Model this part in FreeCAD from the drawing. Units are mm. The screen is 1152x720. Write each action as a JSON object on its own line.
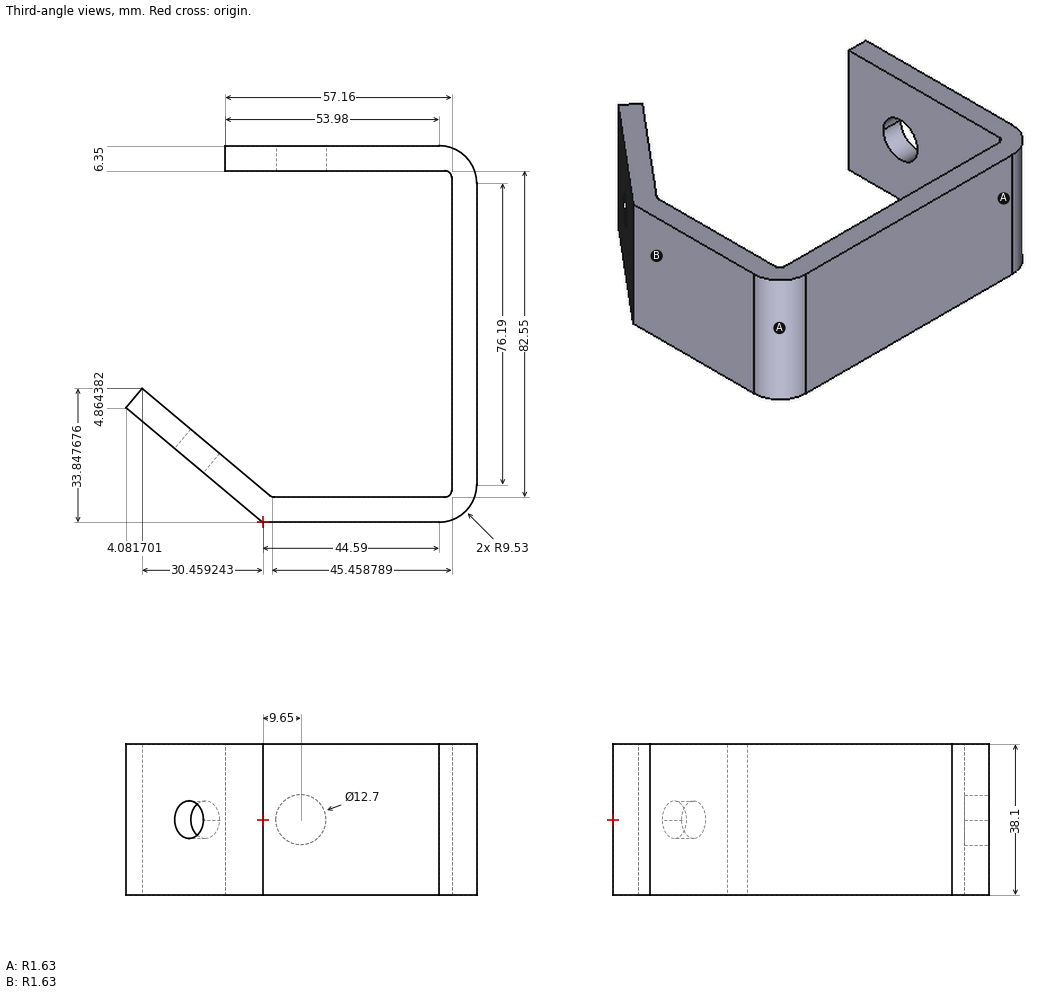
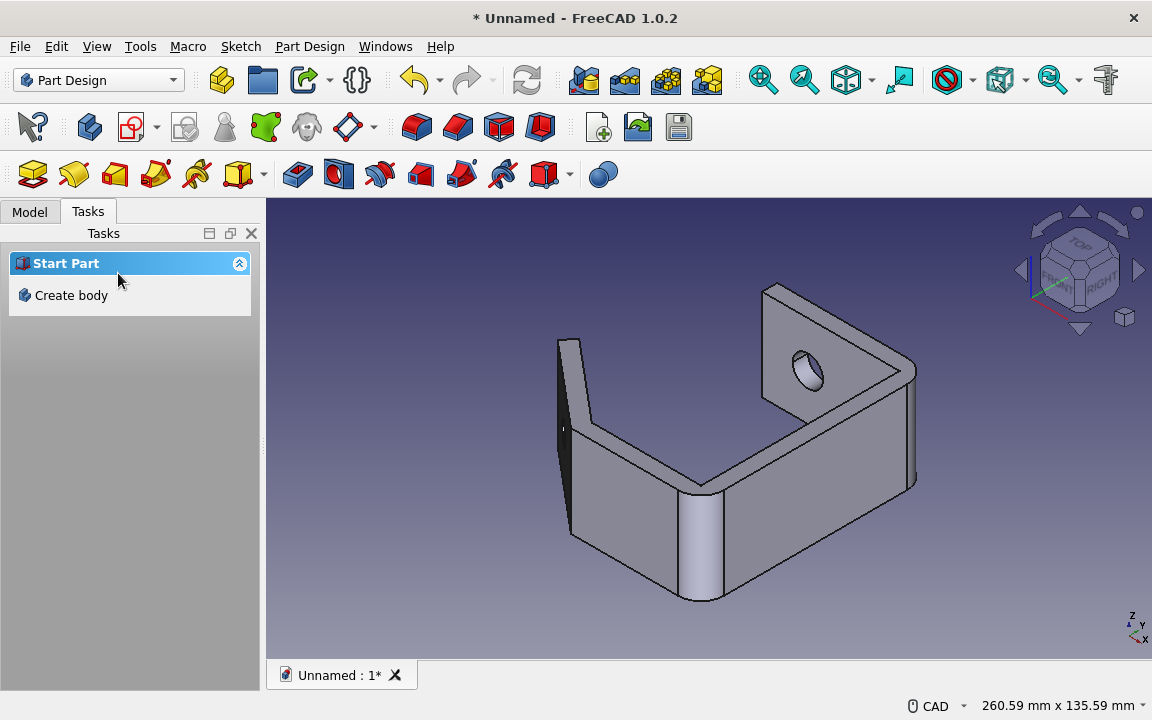
{"action": "key", "text": "2"}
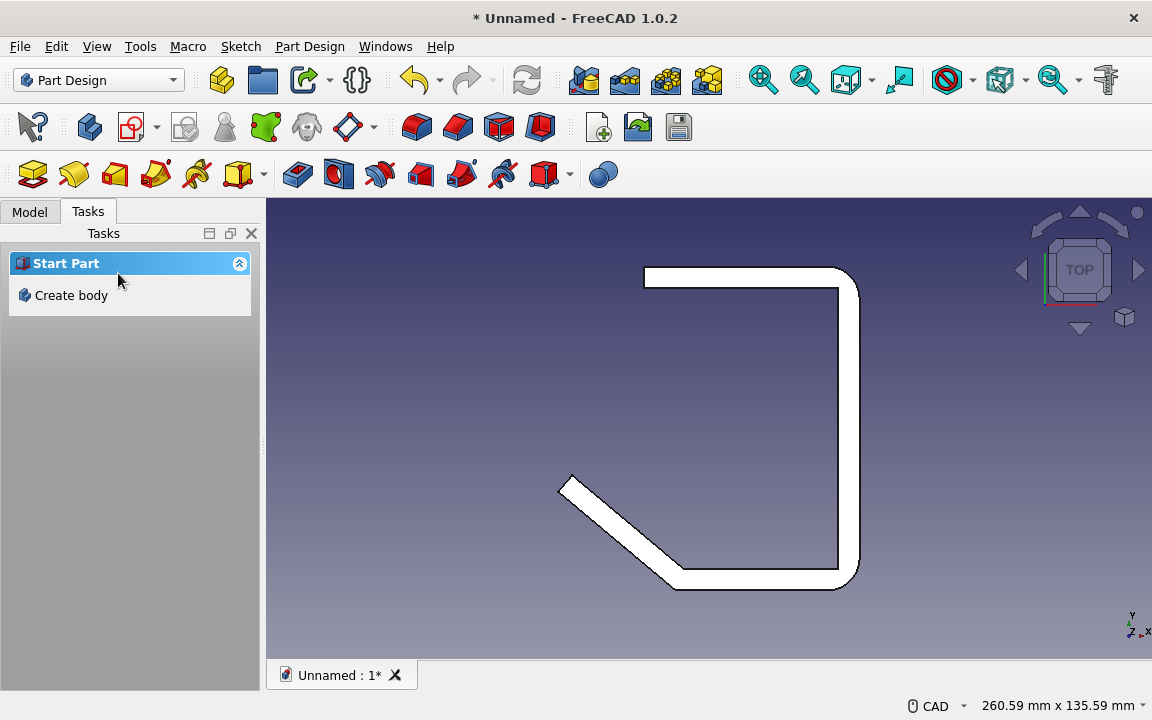
{"action": "key", "text": "1"}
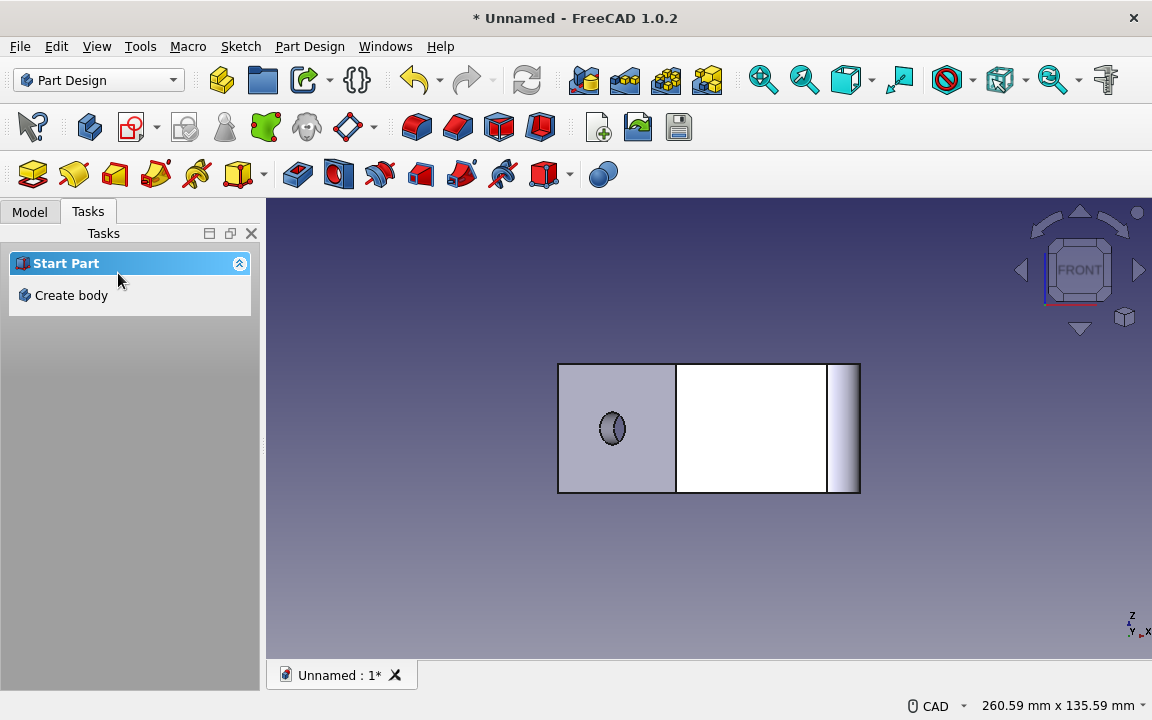
{"action": "key", "text": "v f"}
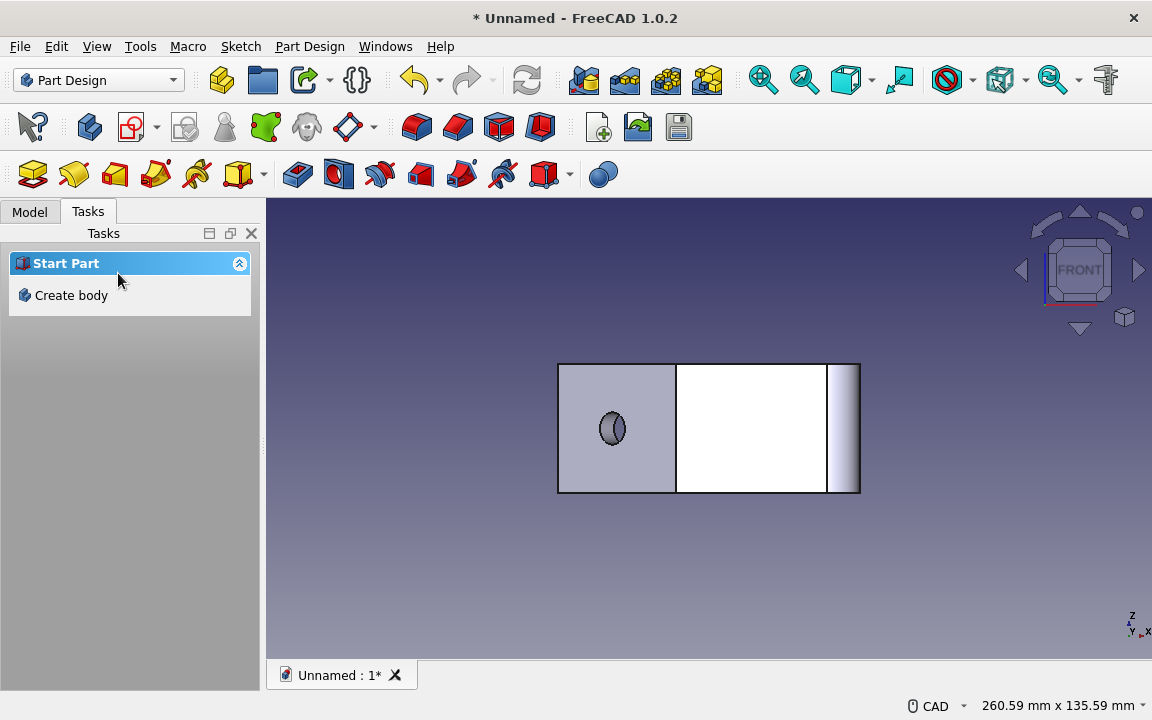
{"action": "key", "text": "3"}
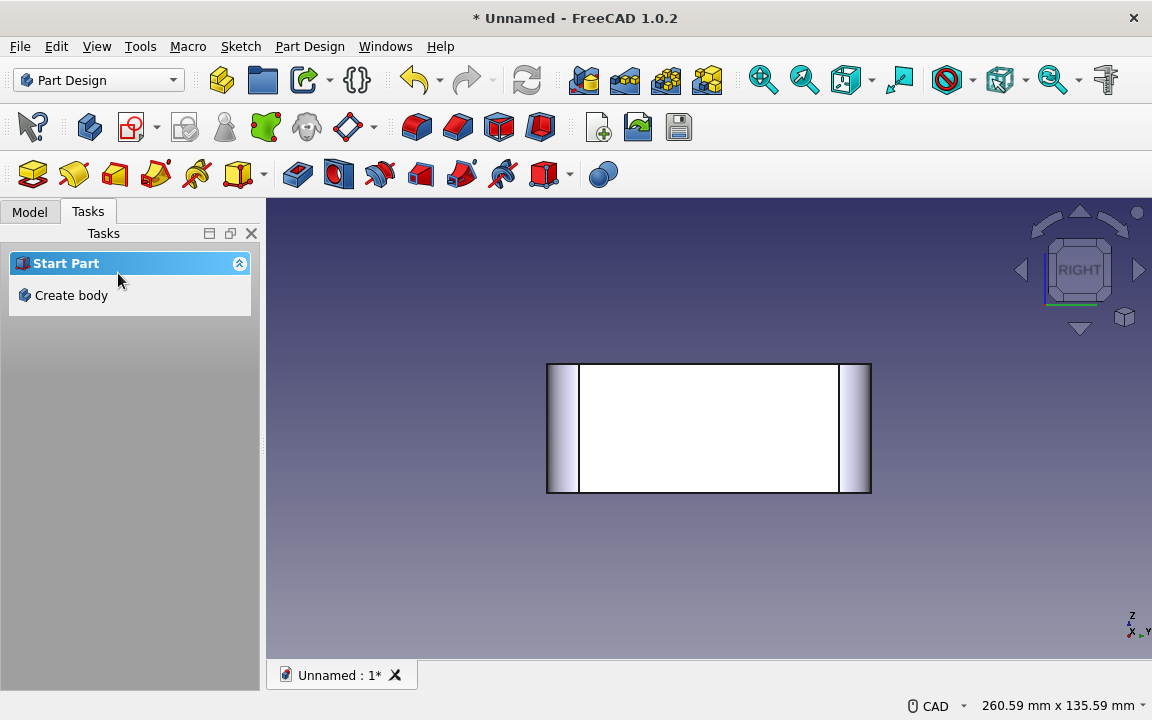
{"action": "key", "text": "v f"}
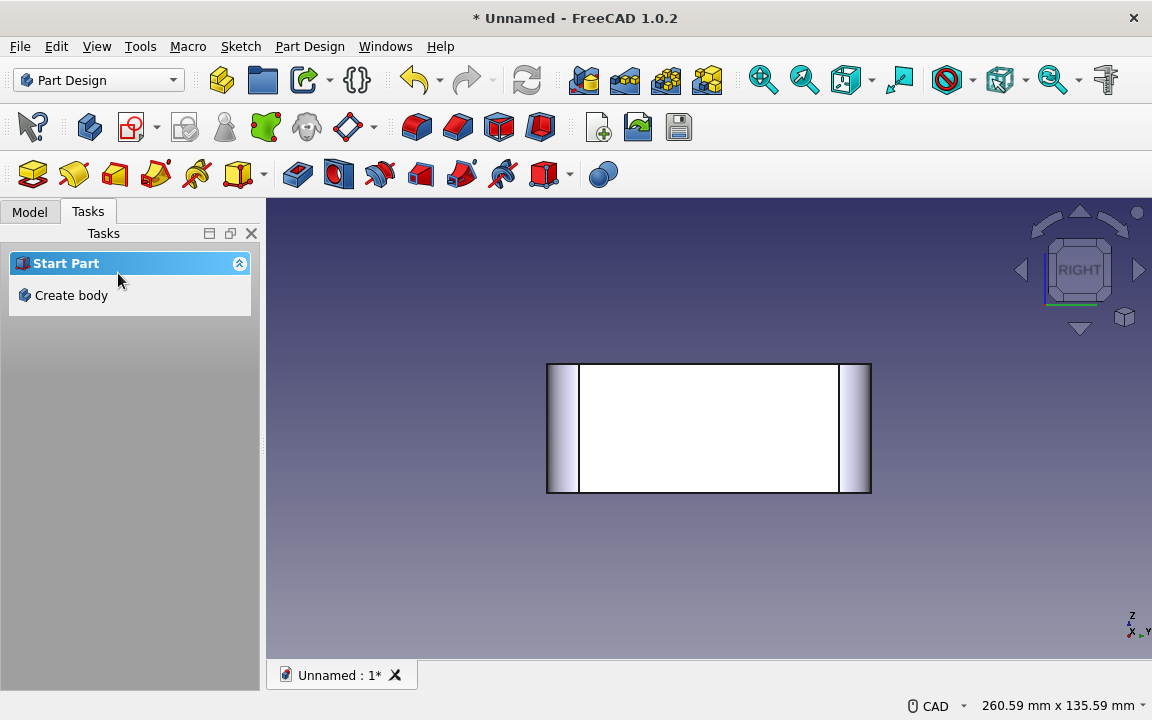
{"action": "key", "text": "5"}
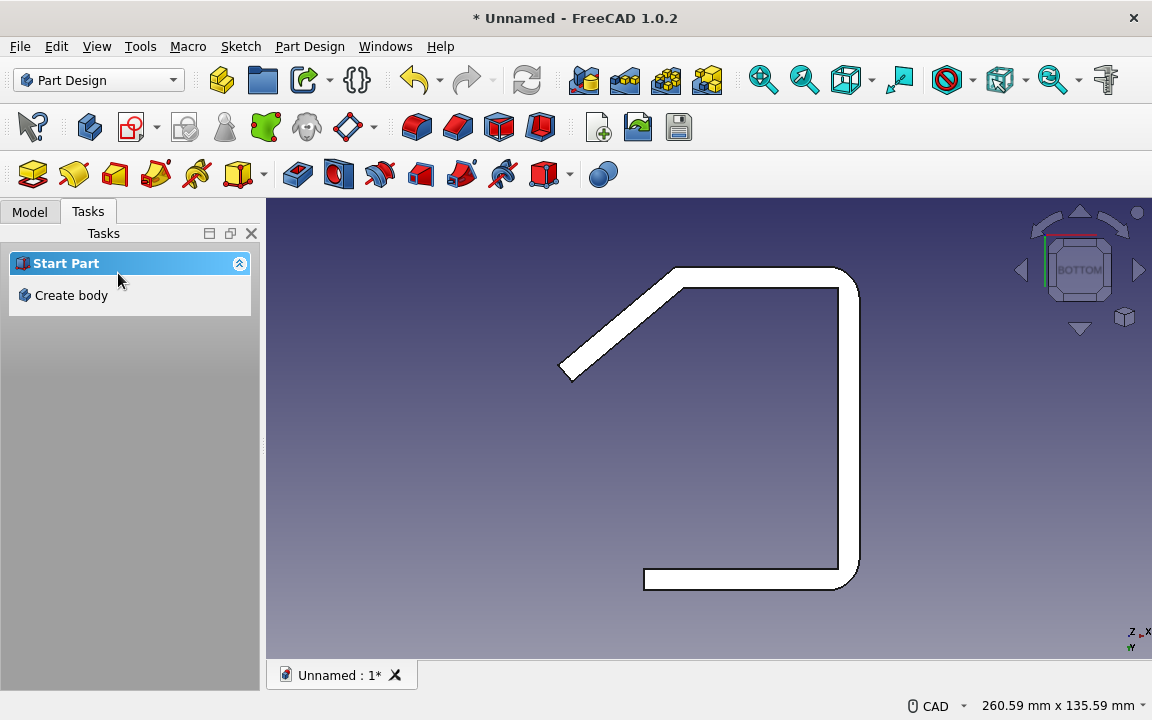
{"action": "key", "text": "4"}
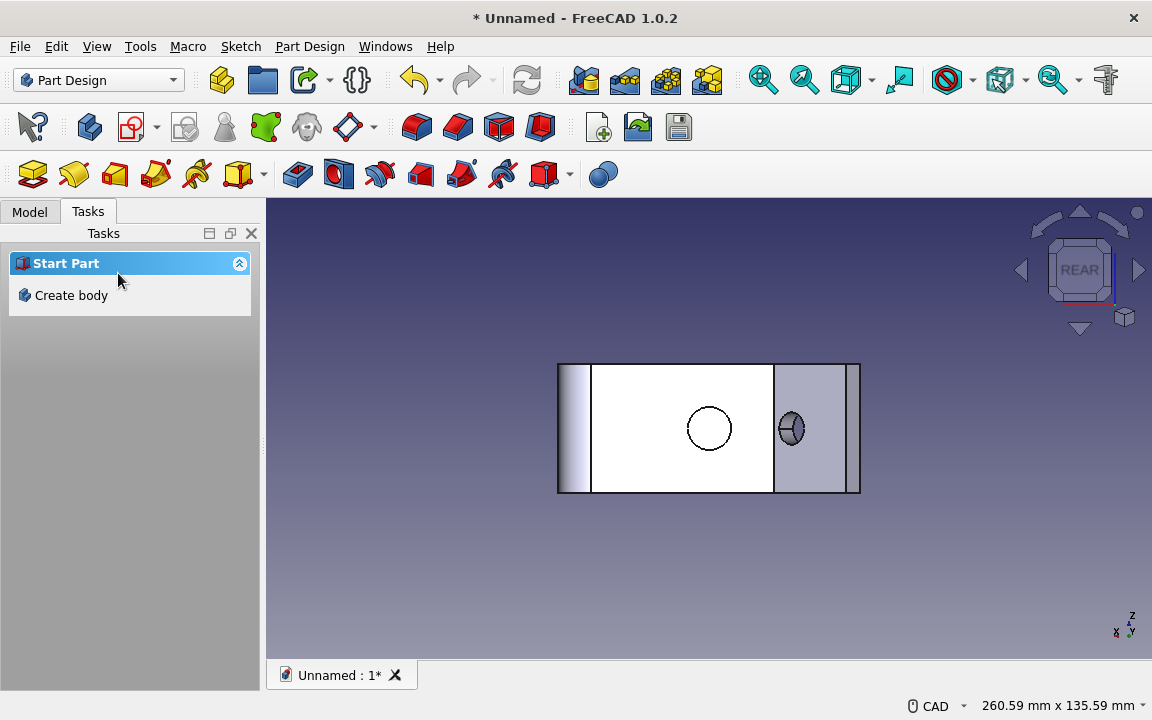
{"action": "key", "text": "v f"}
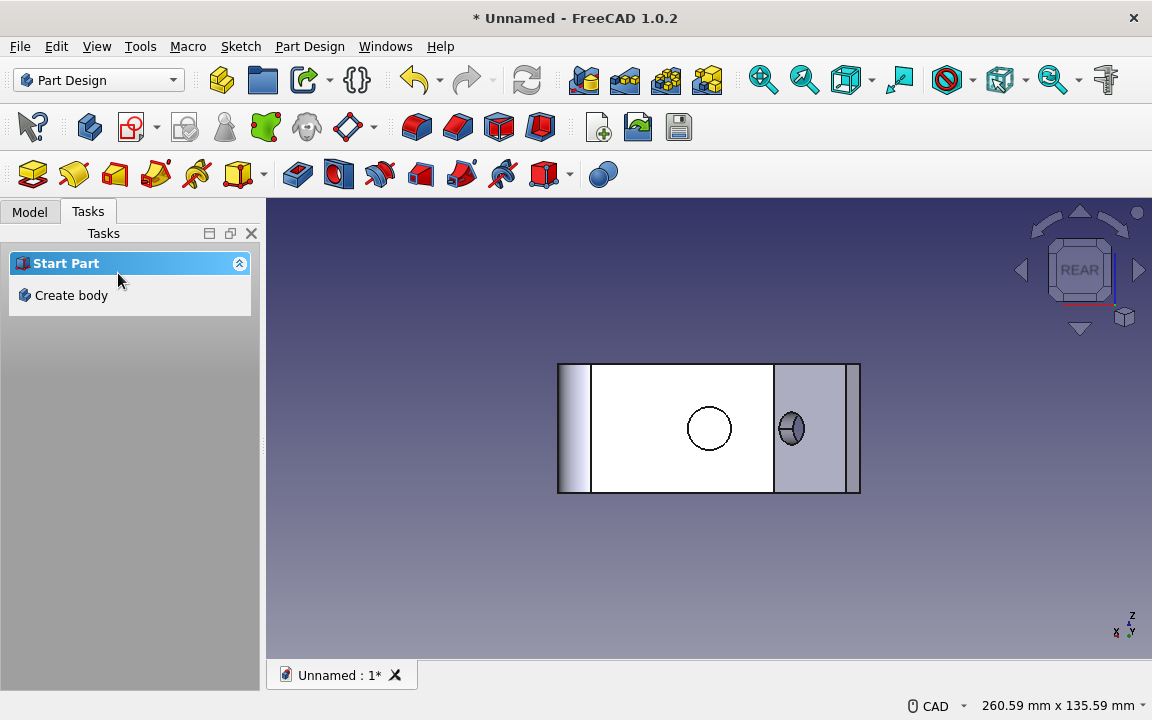
{"action": "key", "text": "6"}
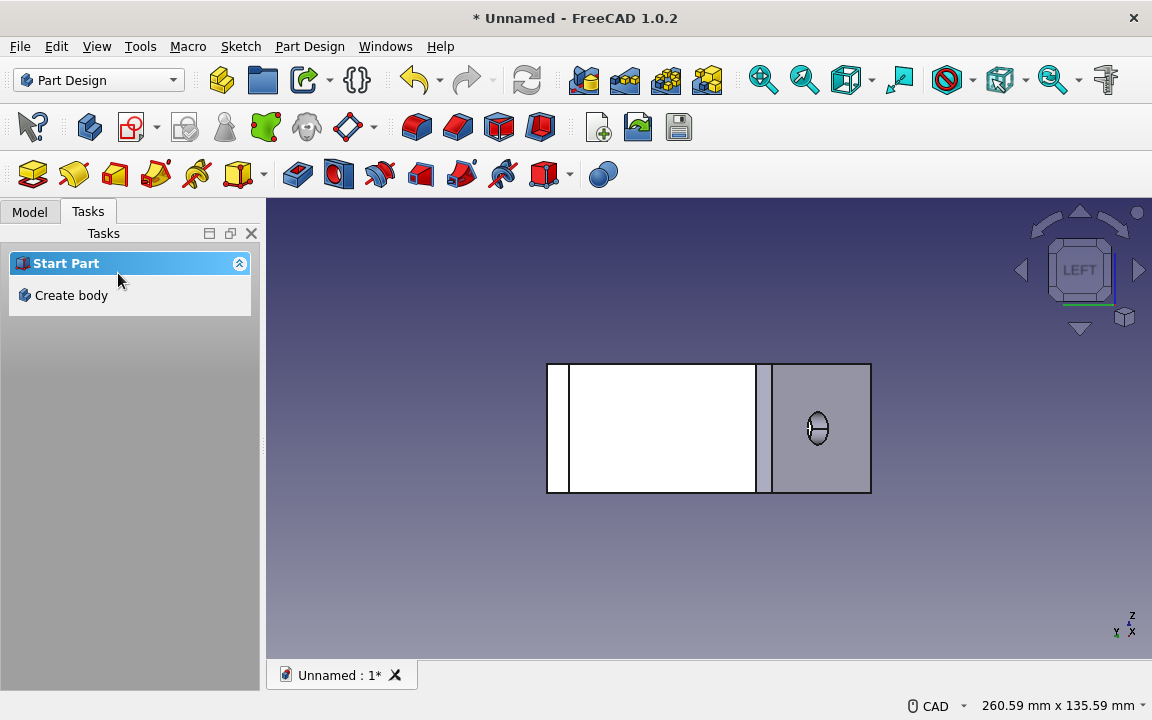
{"action": "key", "text": "v f"}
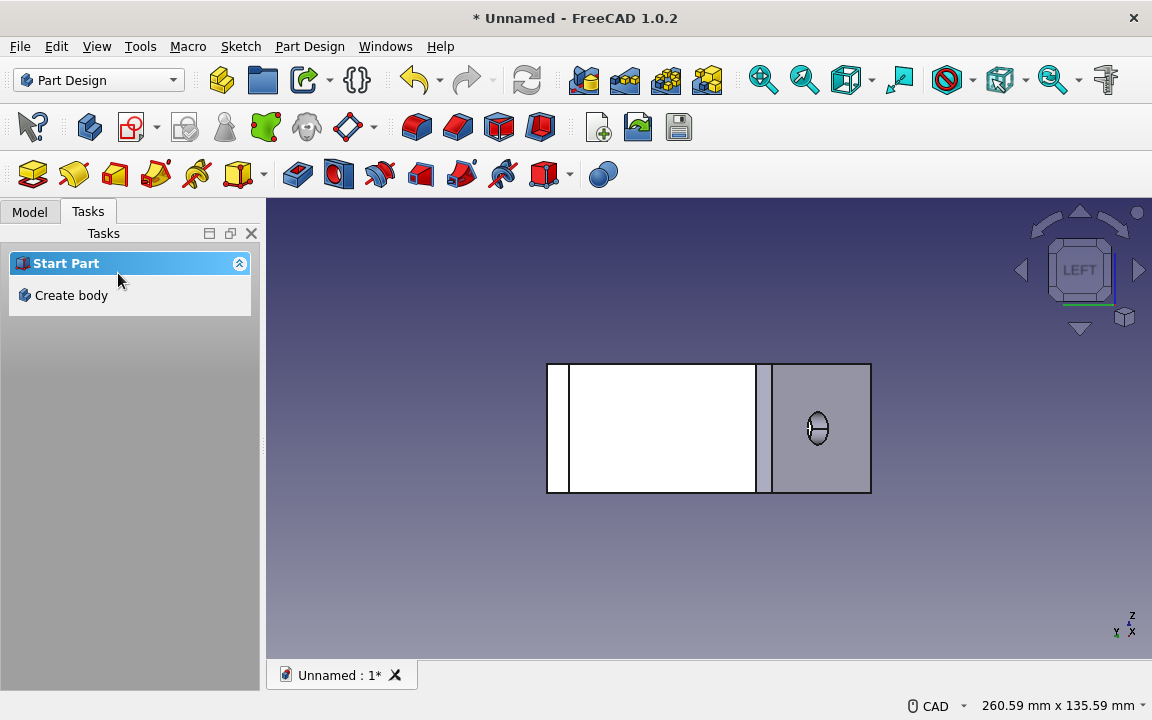
{"action": "key", "text": "v 3"}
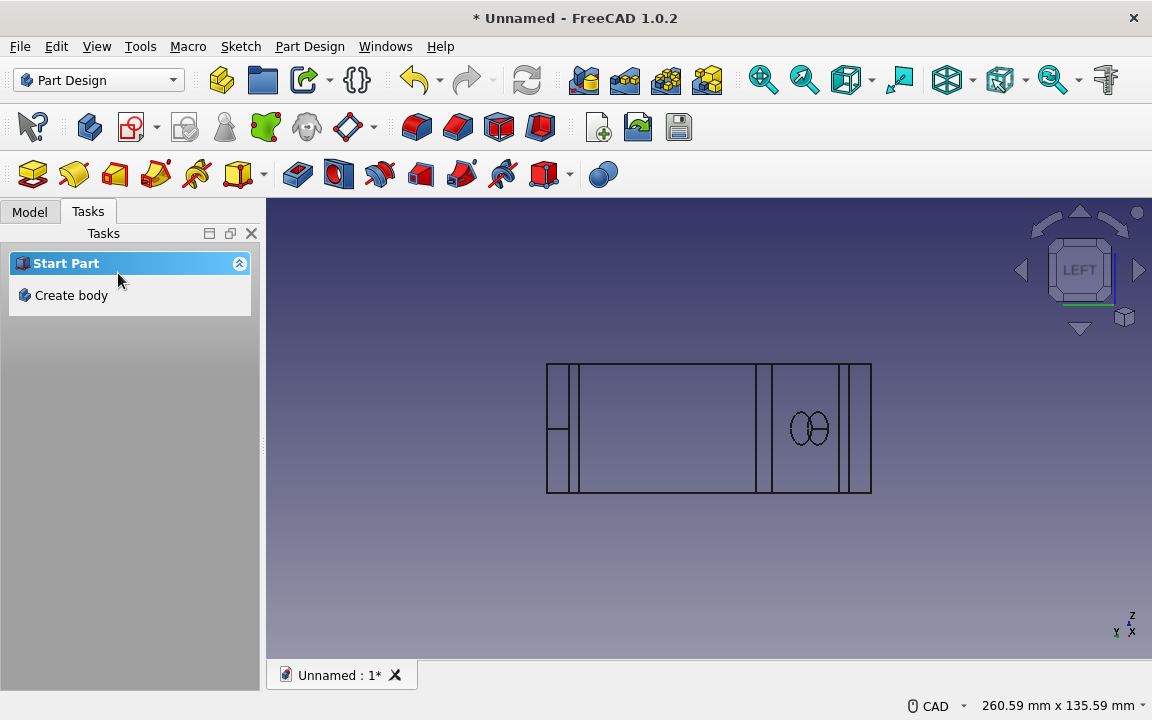
{"action": "key", "text": "0"}